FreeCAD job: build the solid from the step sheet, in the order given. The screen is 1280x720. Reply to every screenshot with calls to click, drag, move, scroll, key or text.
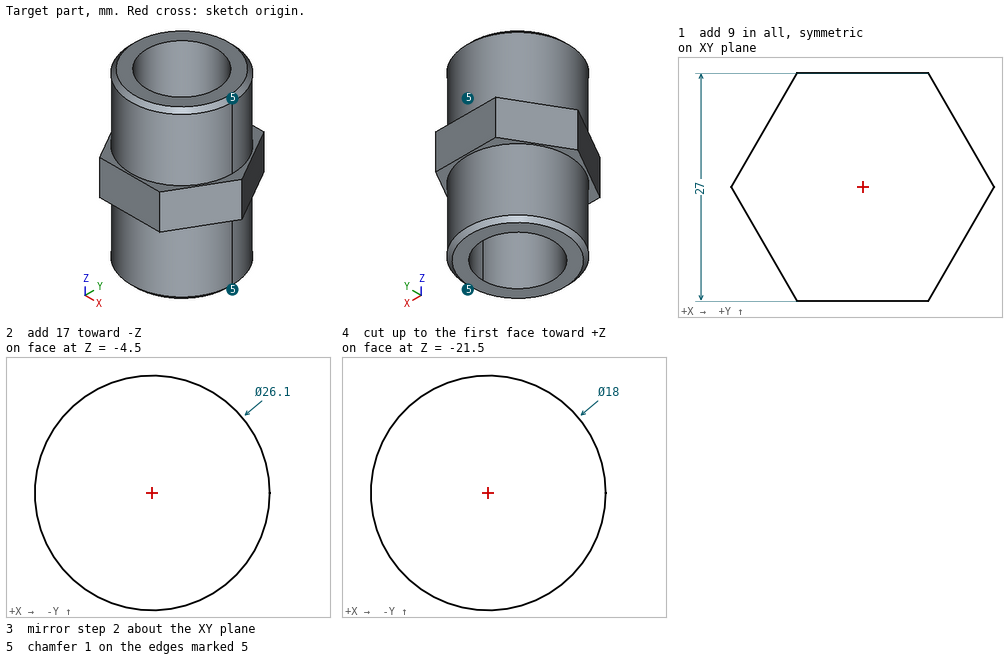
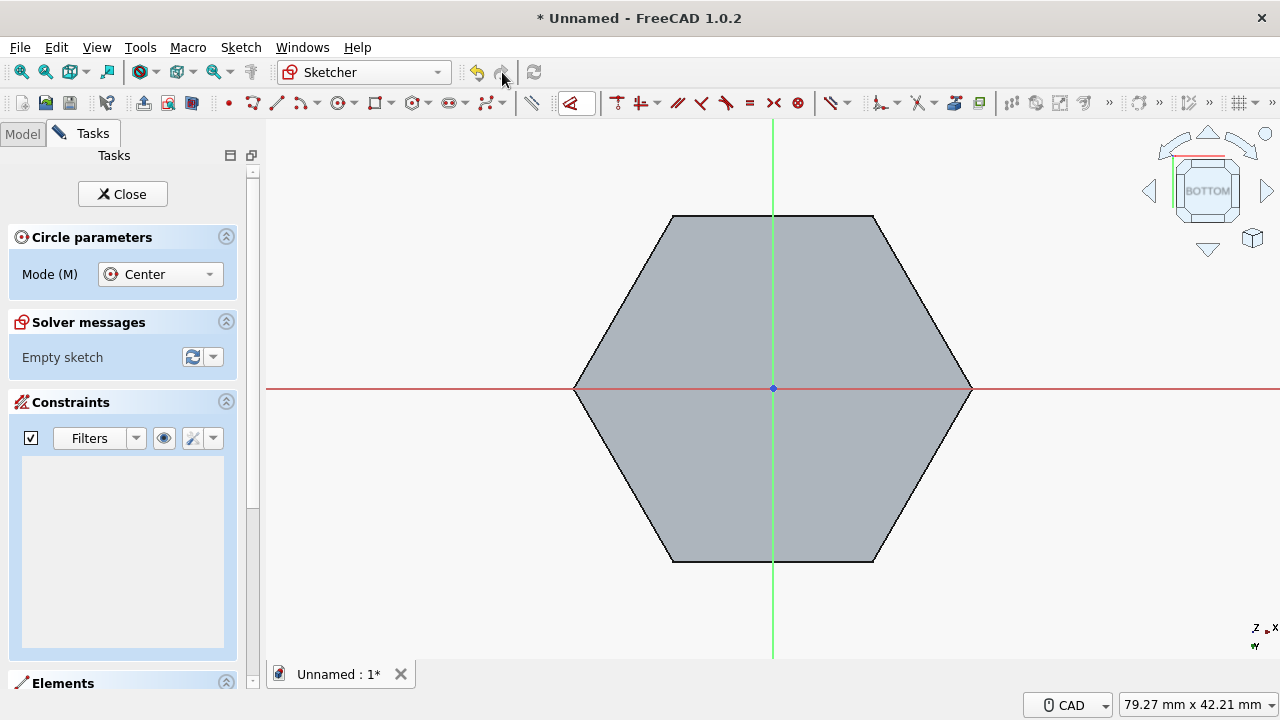
click(773, 389)
move(891, 271)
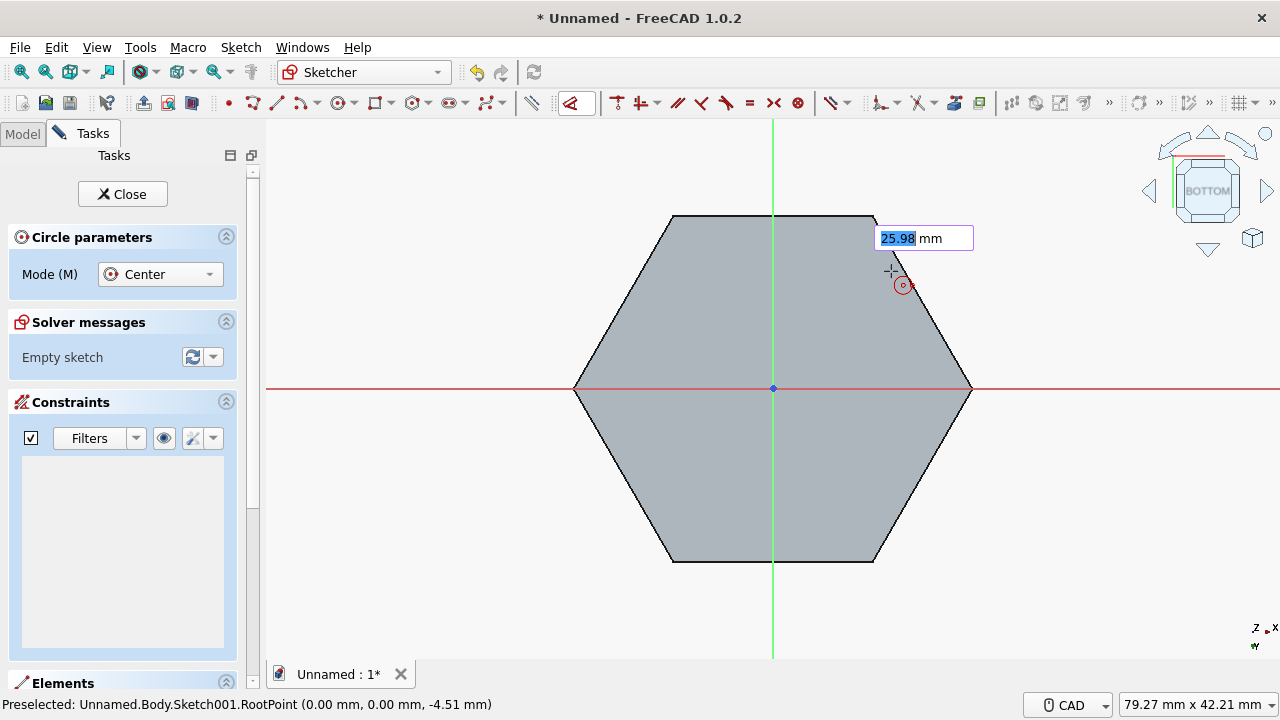
text(26.1)
key(Return)
key(Escape)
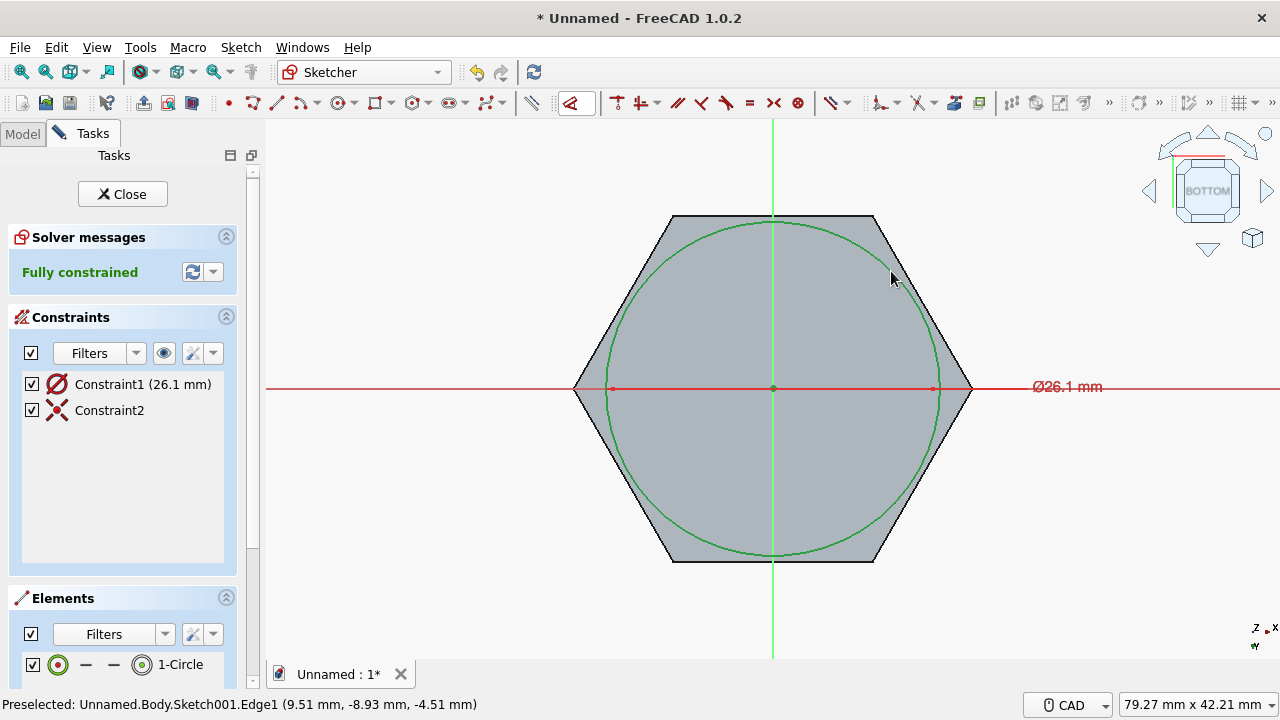
click(123, 194)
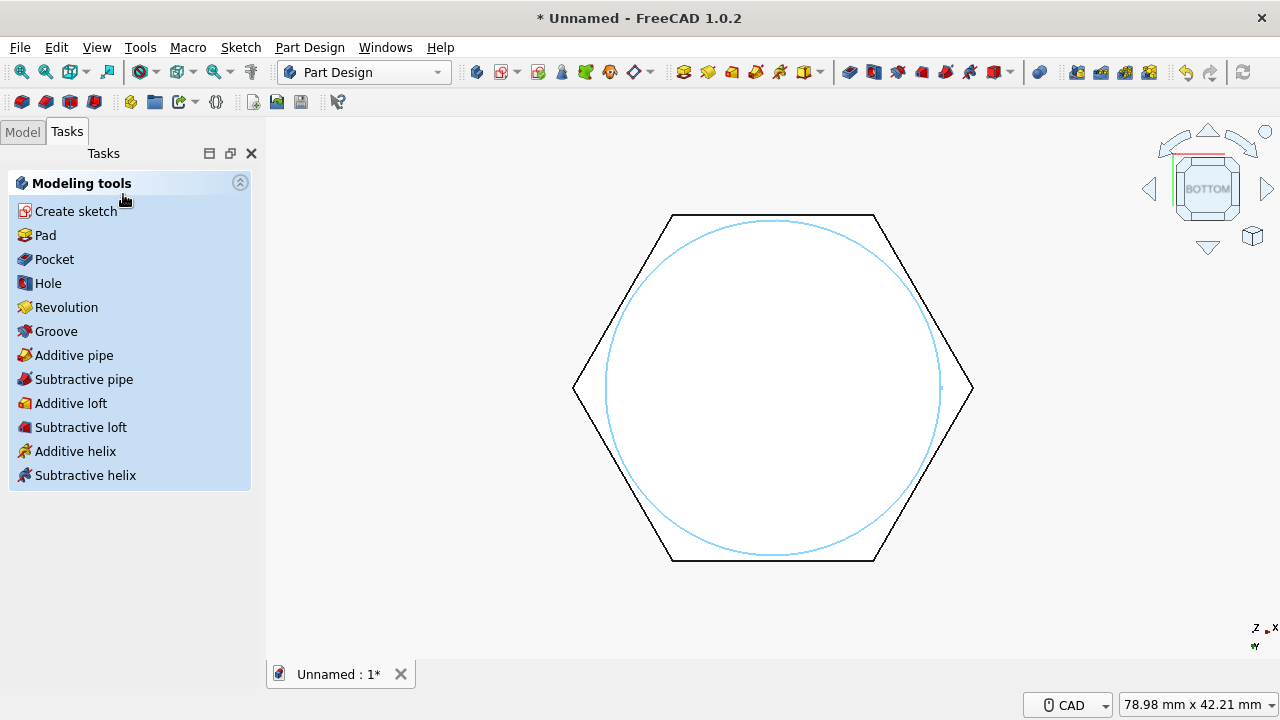
click(684, 72)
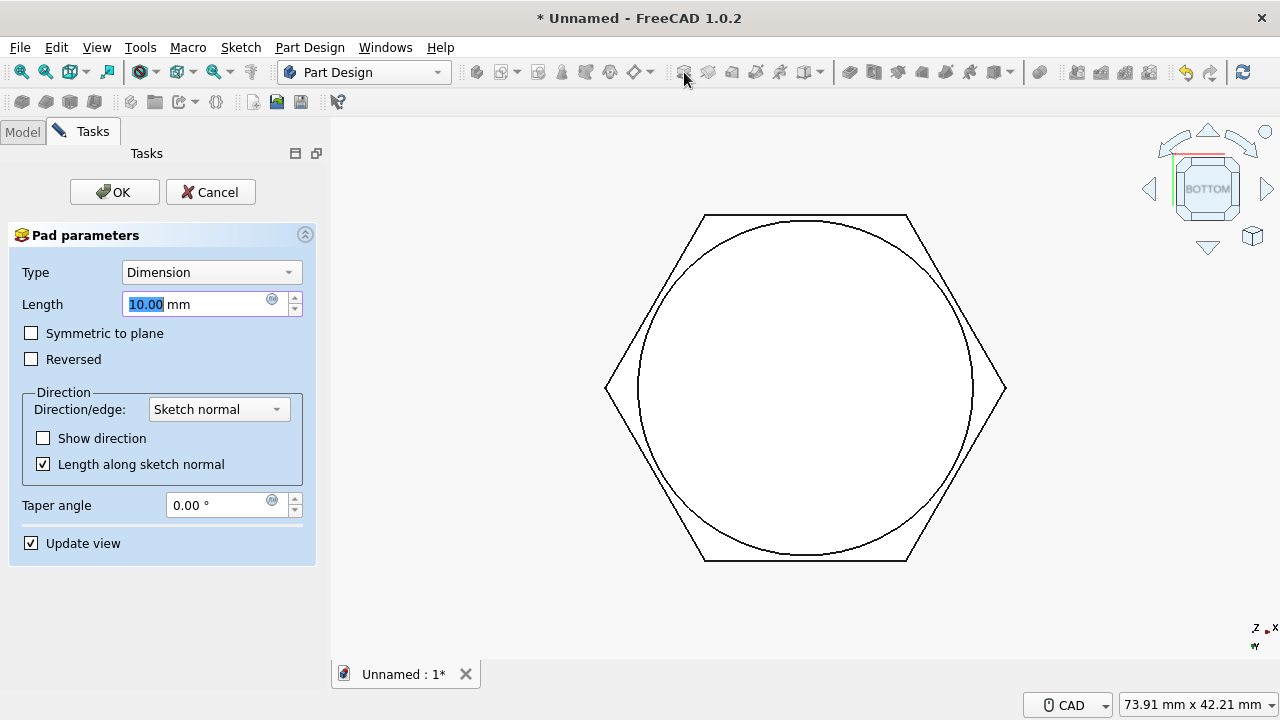
text(17)
key(Tab)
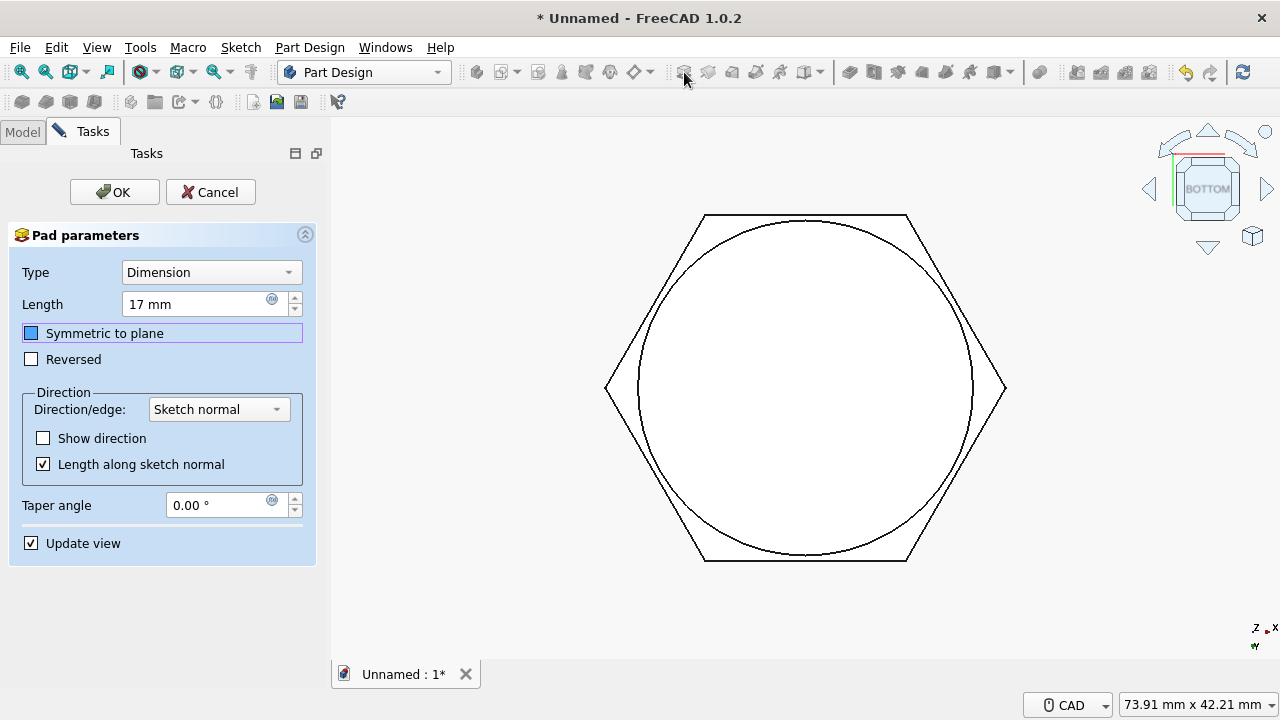
click(115, 192)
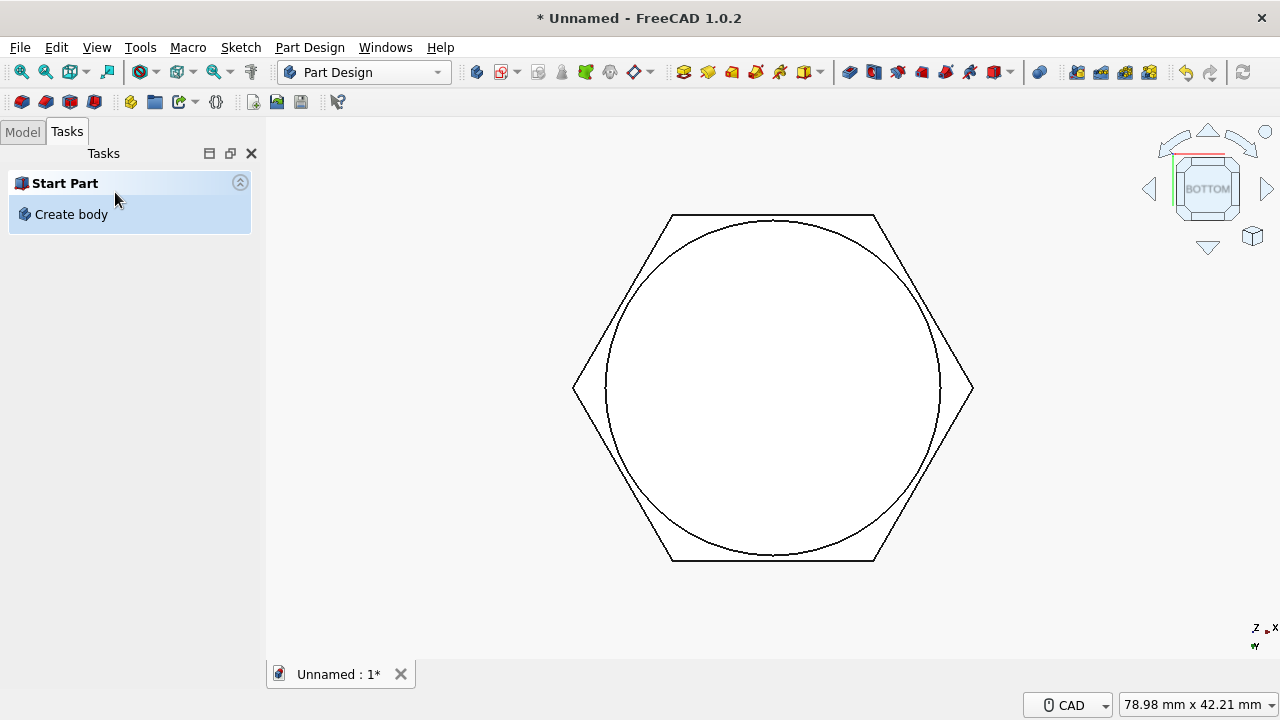
click(23, 131)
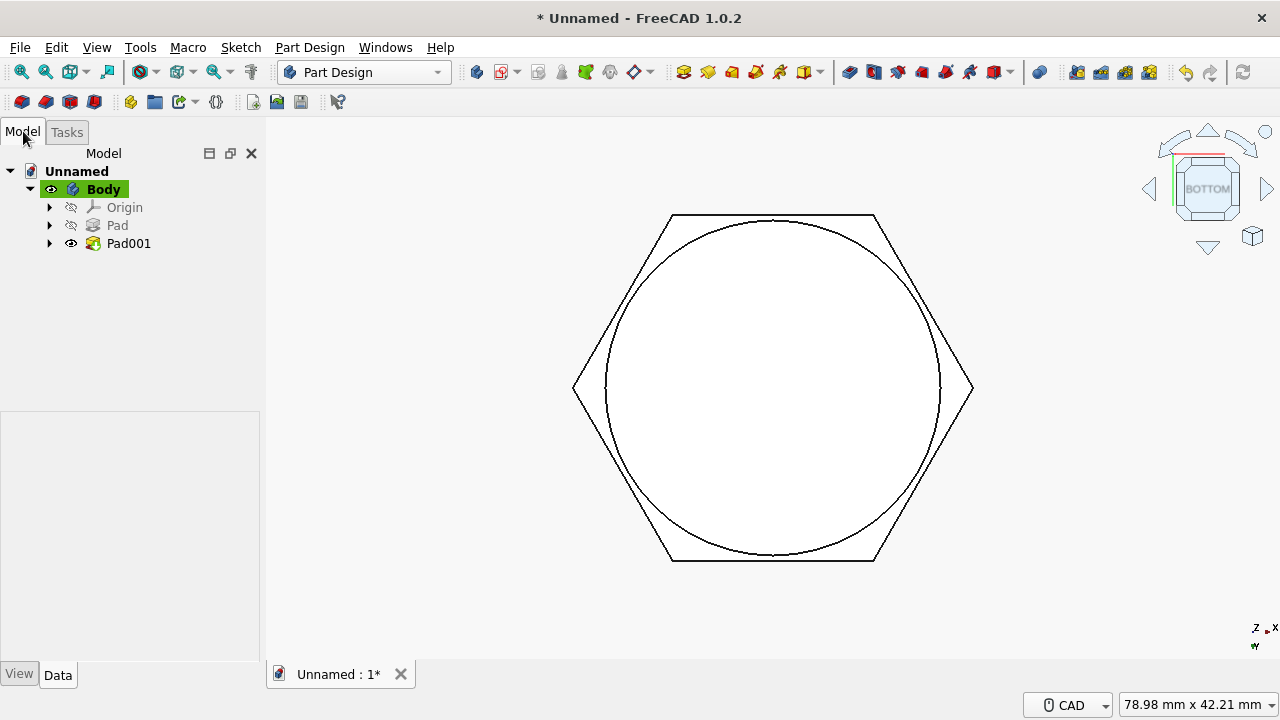
click(116, 243)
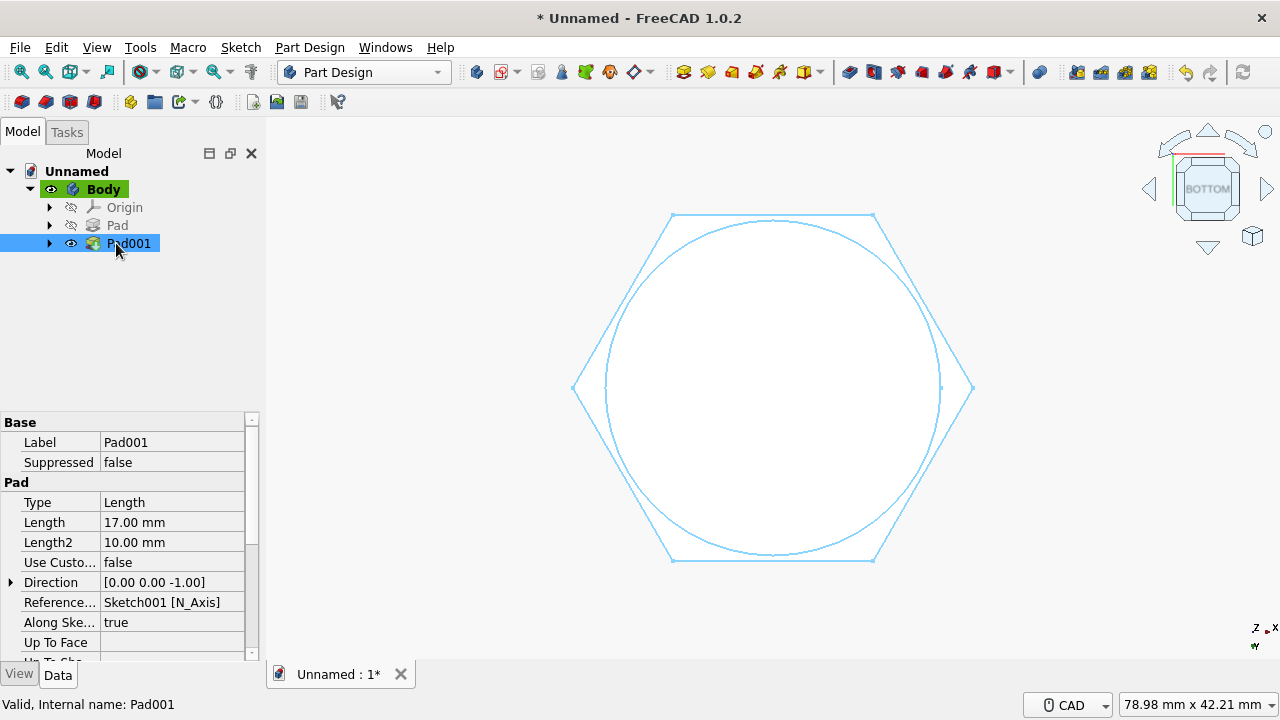
click(1078, 72)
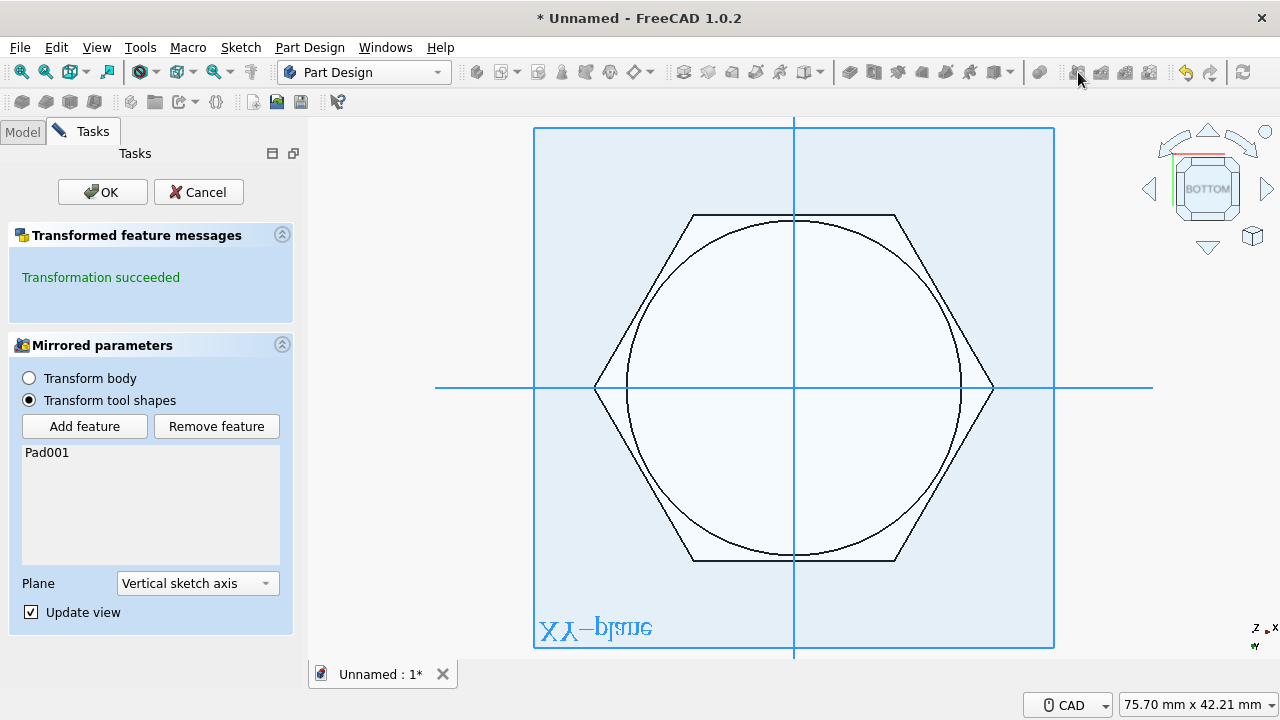
click(198, 584)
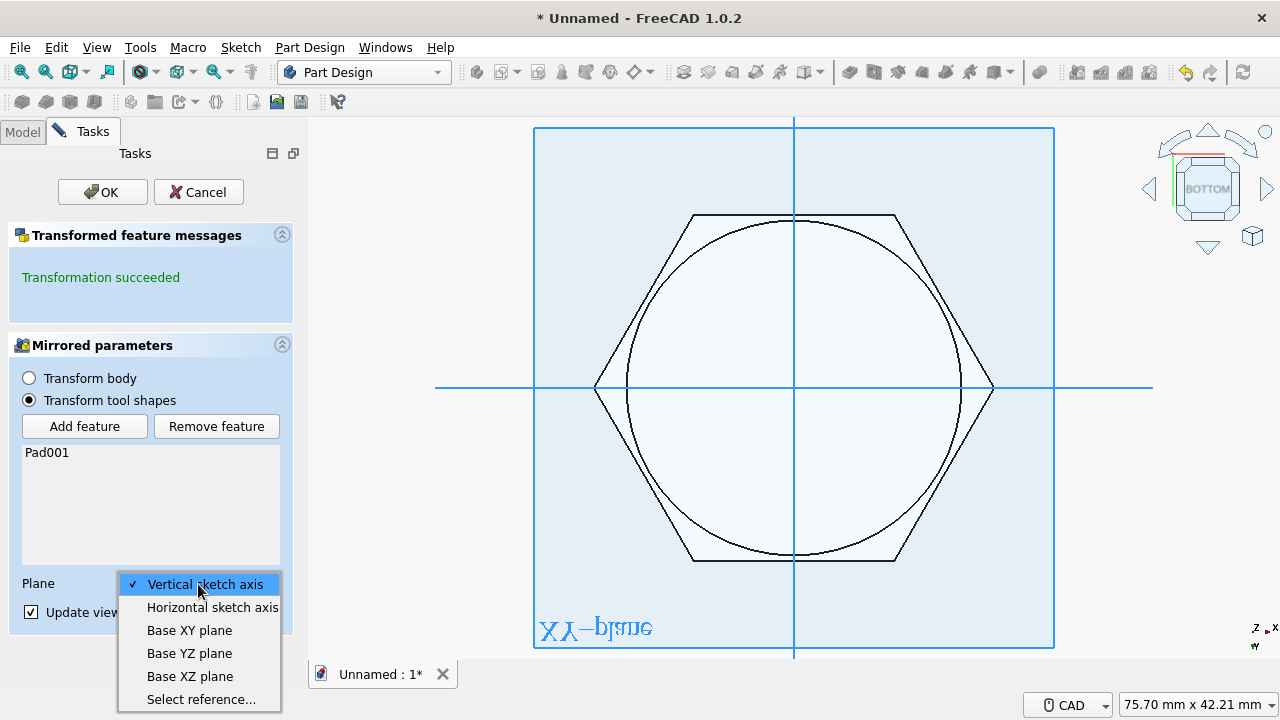
click(198, 630)